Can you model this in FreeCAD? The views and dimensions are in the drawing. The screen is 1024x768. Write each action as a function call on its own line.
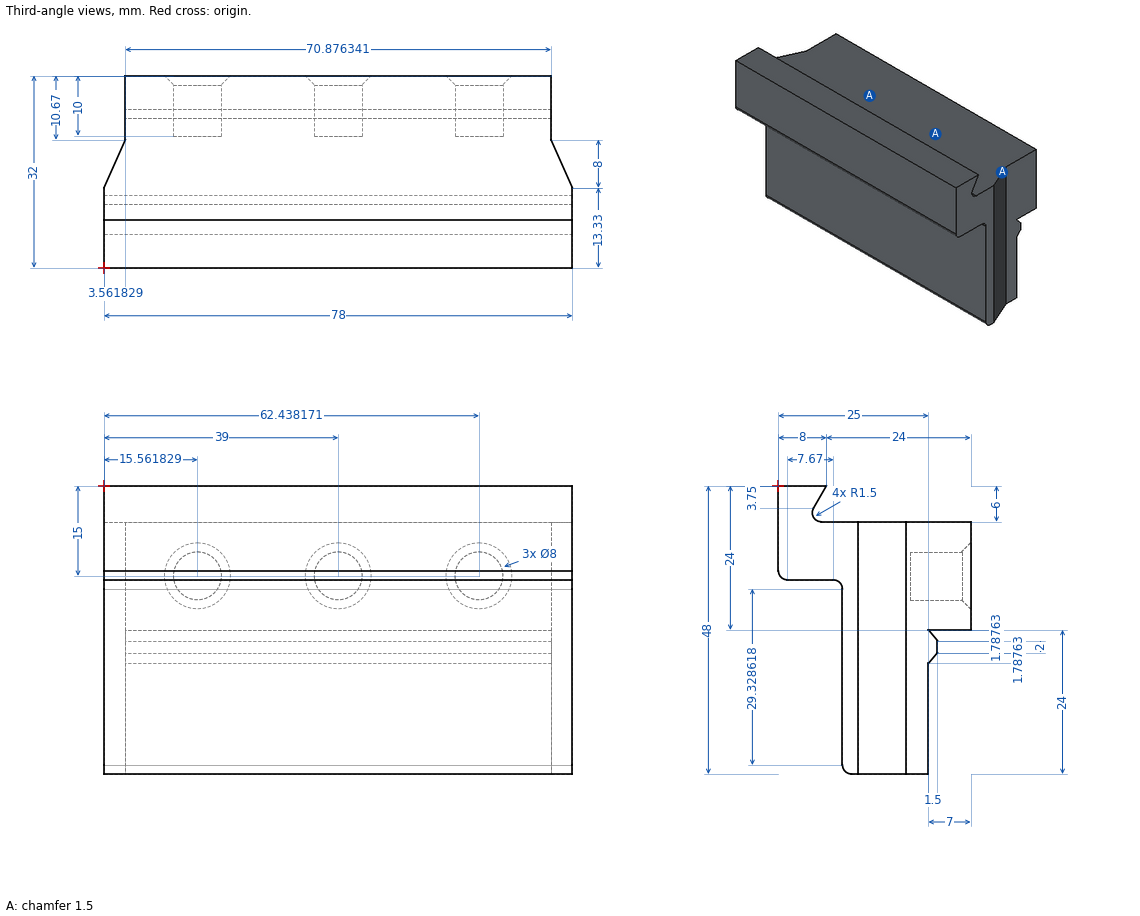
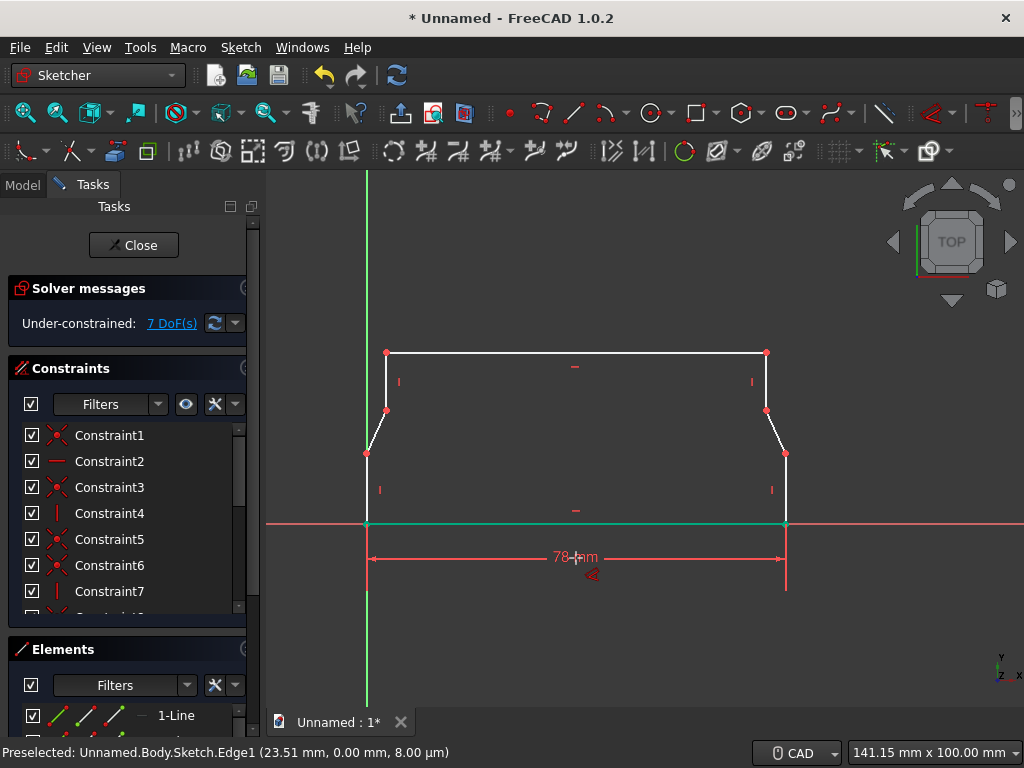
click(780, 441)
click(820, 433)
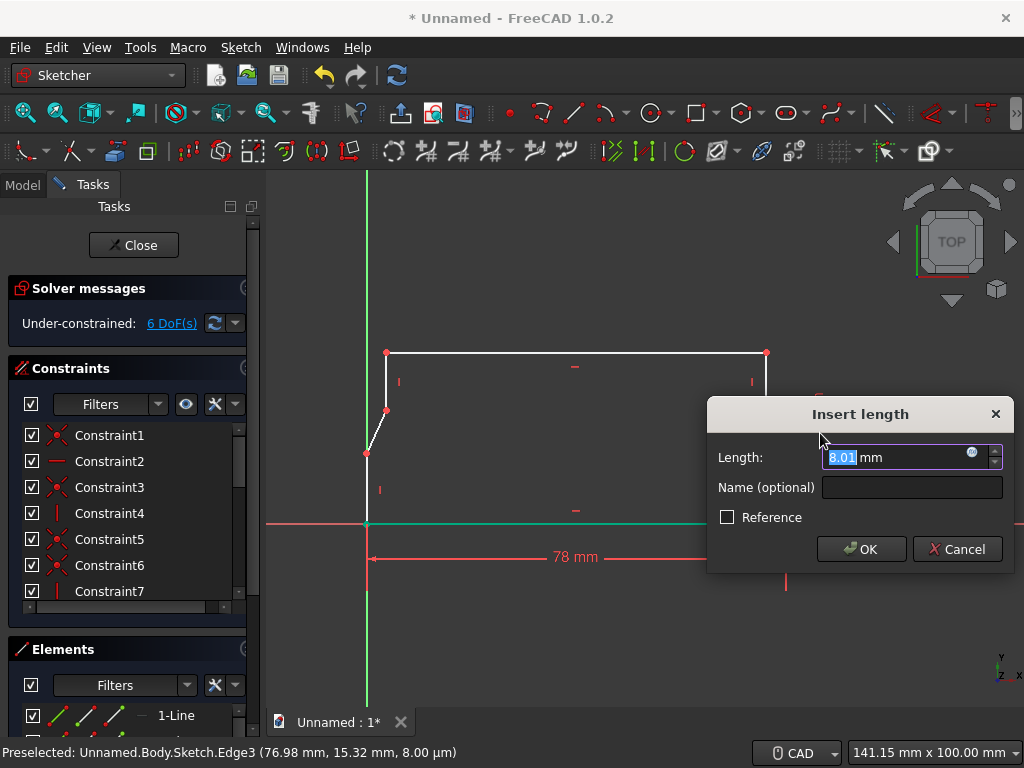
text(8)
key(Return)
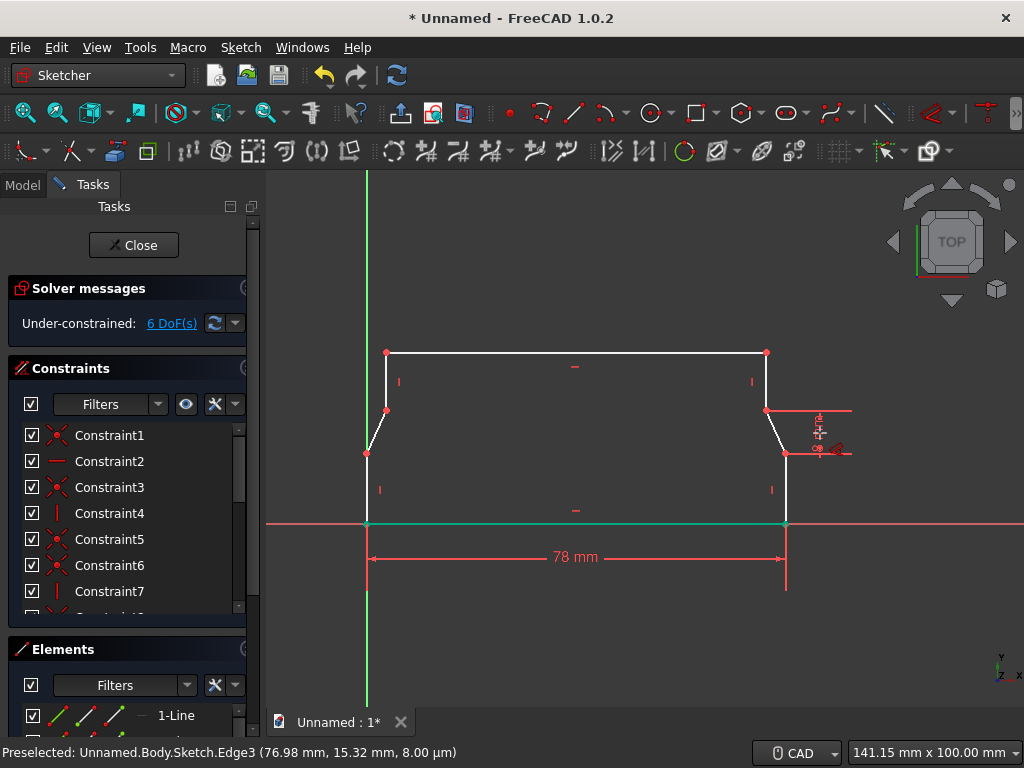
click(380, 424)
click(333, 433)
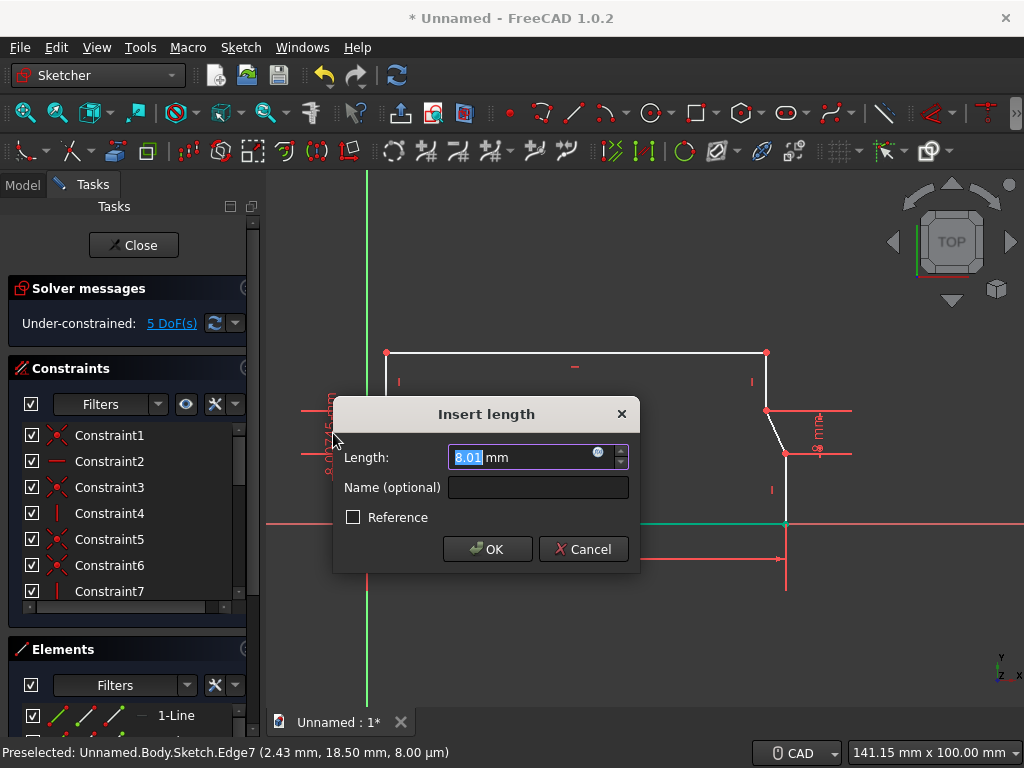
text(8)
key(Return)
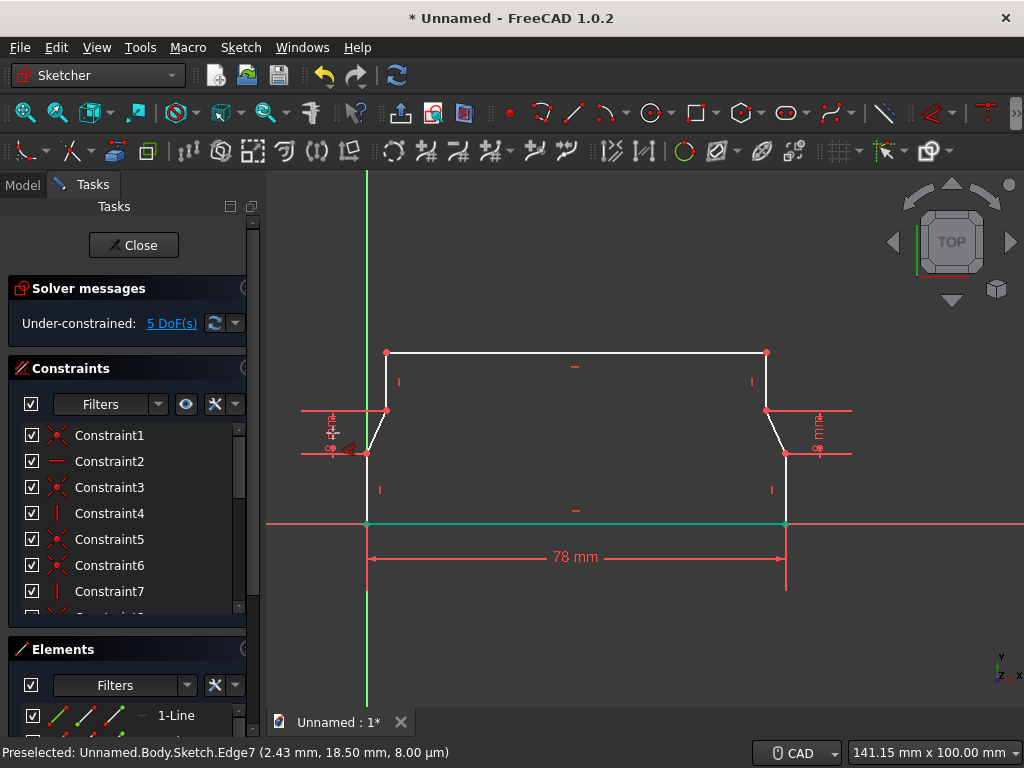
click(766, 353)
click(333, 399)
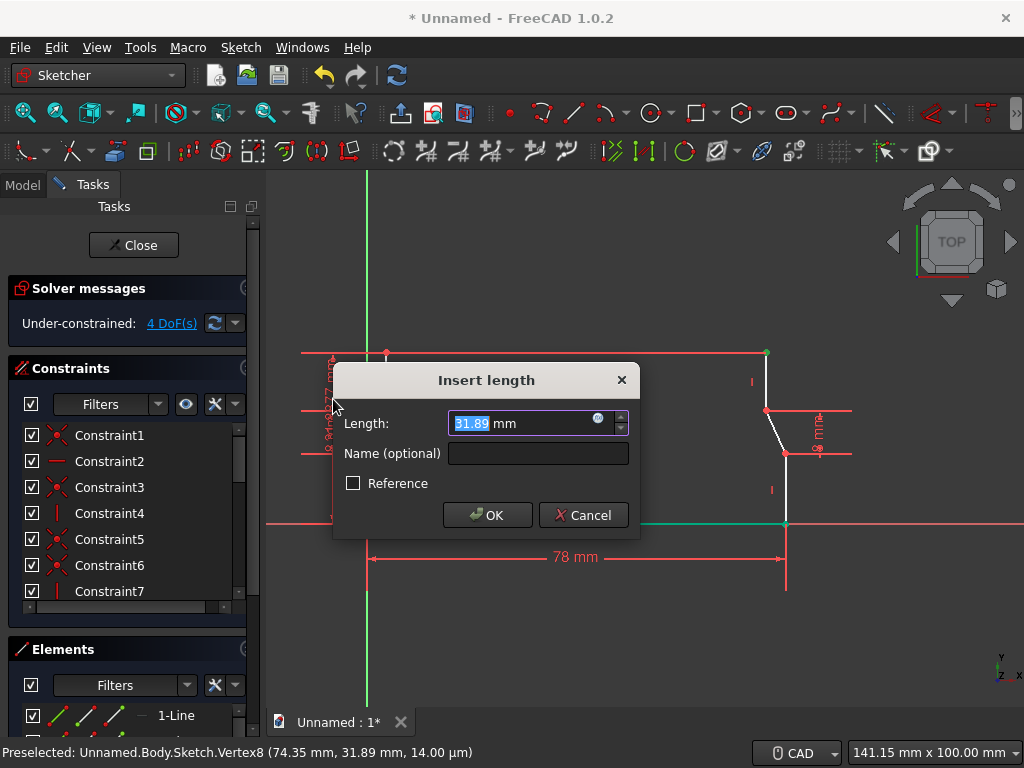
text(32)
key(Return)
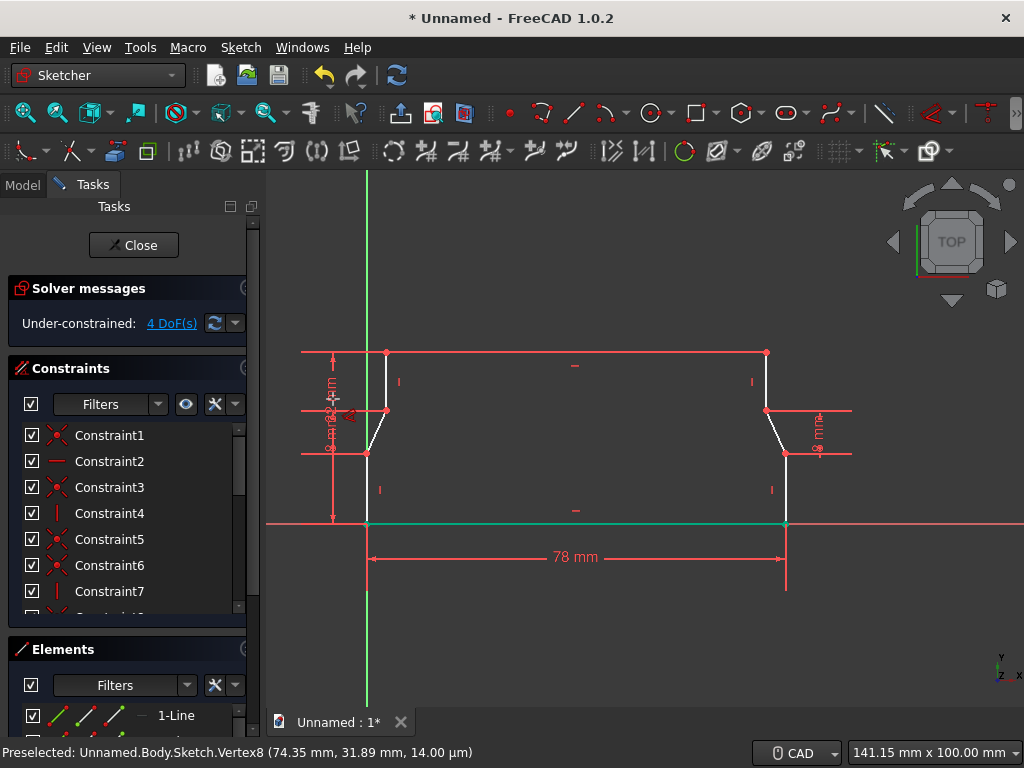
click(786, 503)
click(820, 489)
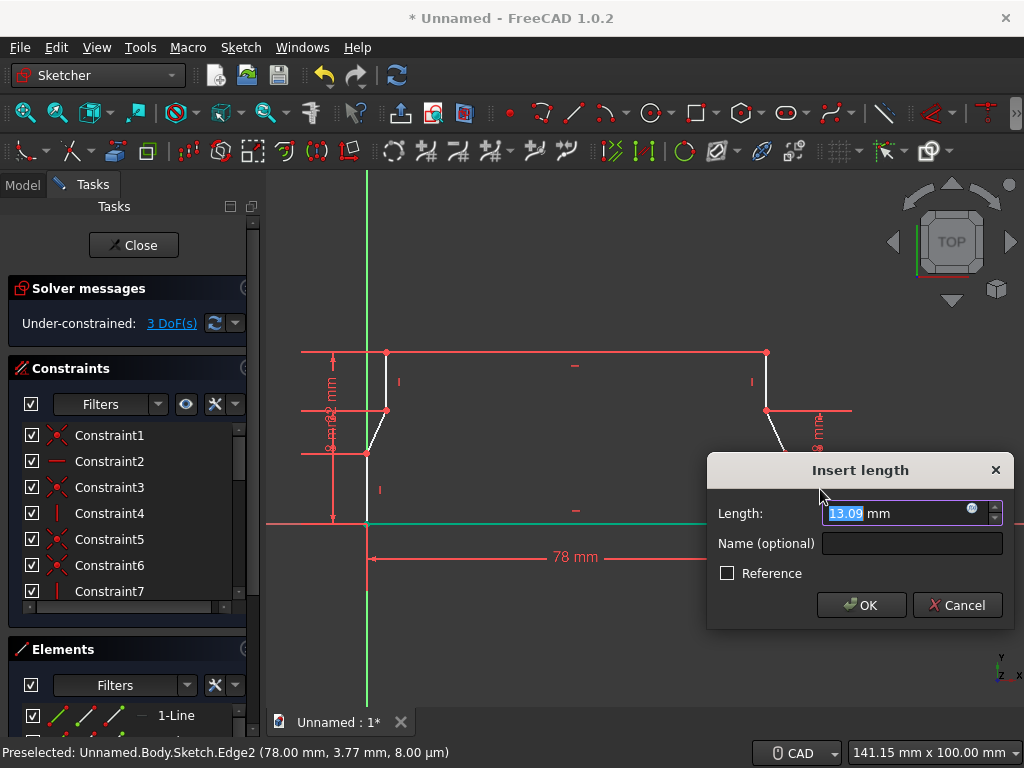
text(13.33)
key(Return)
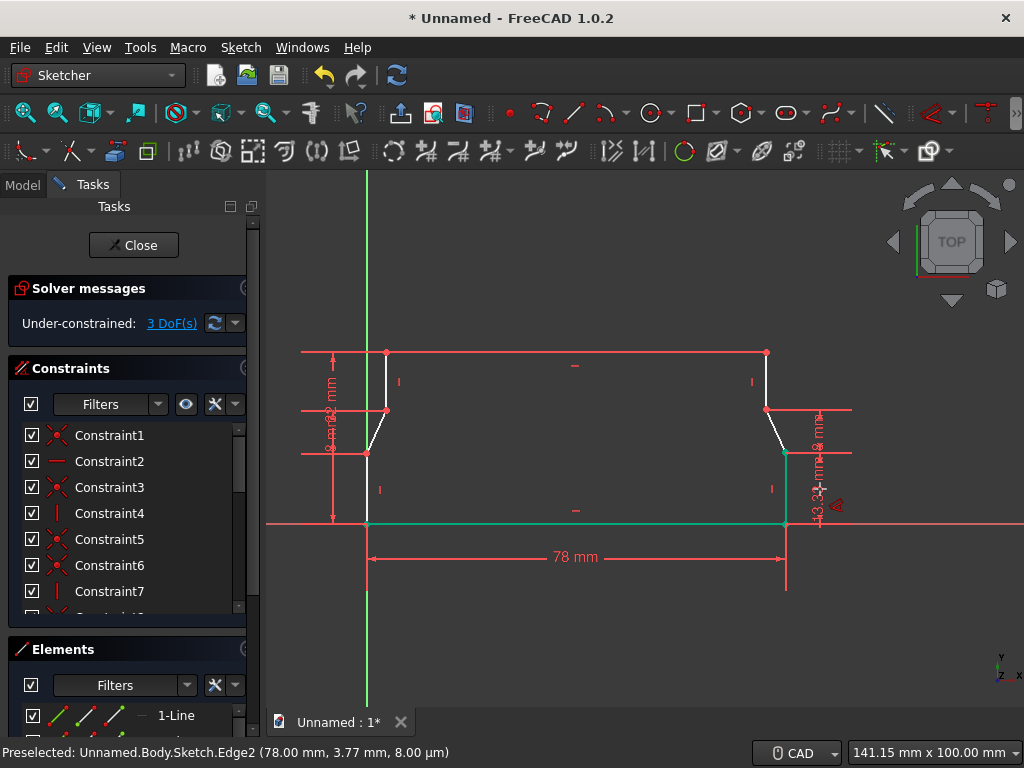
click(386, 370)
click(352, 368)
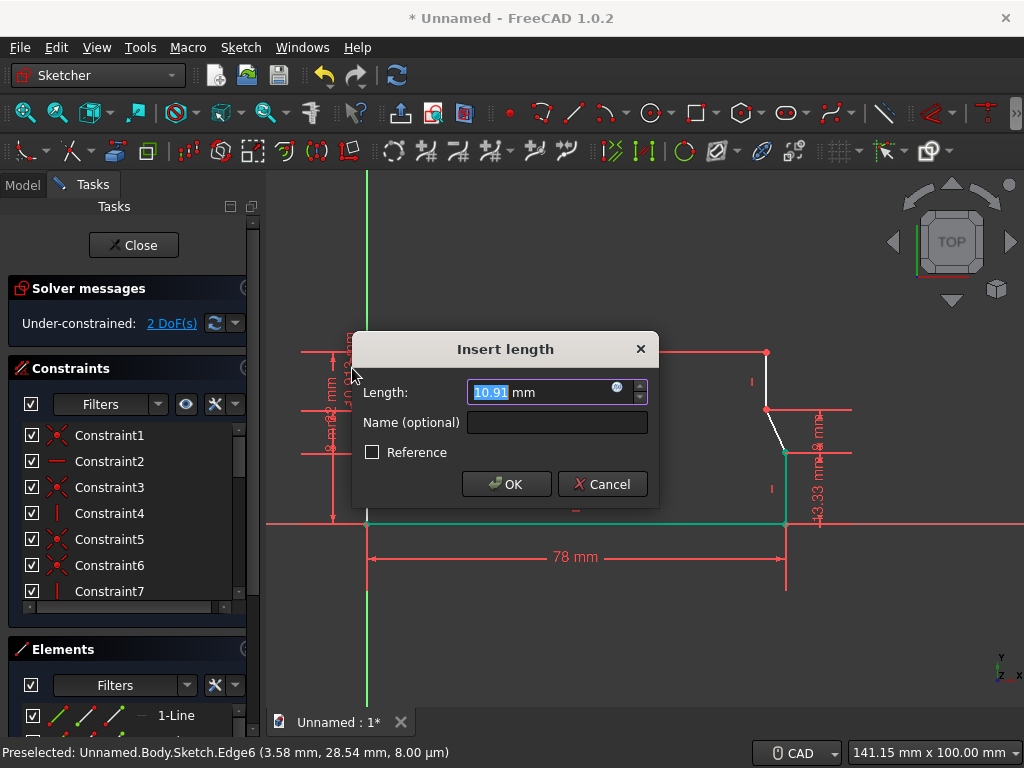
text(10.67)
key(Return)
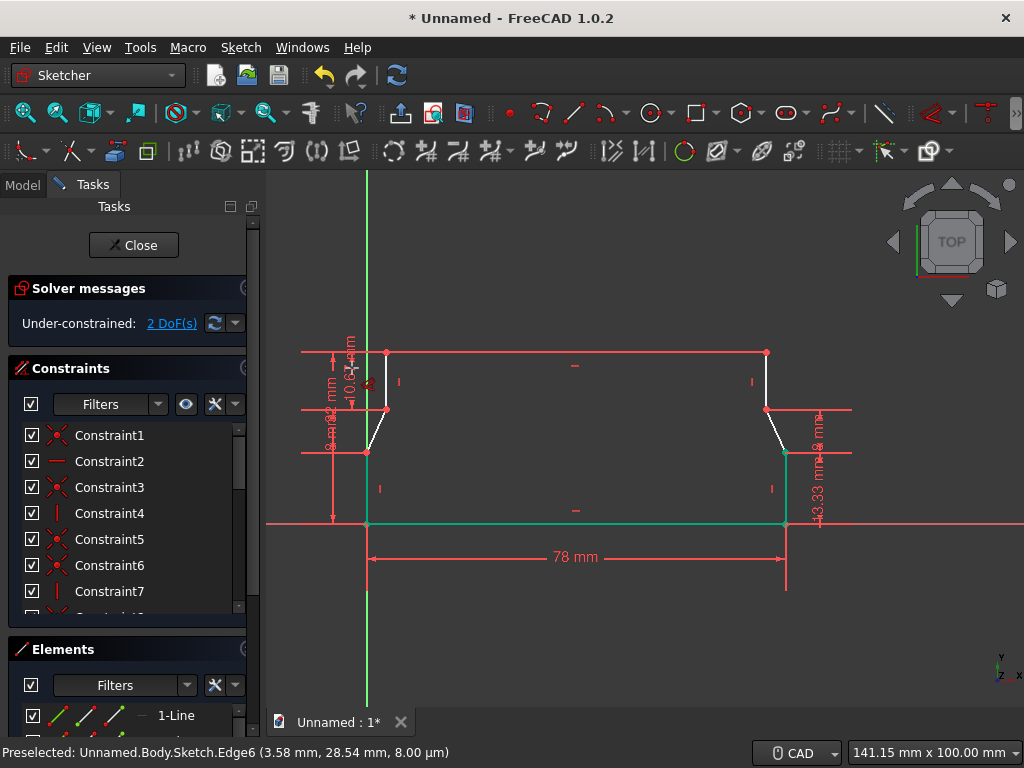
click(652, 352)
click(576, 318)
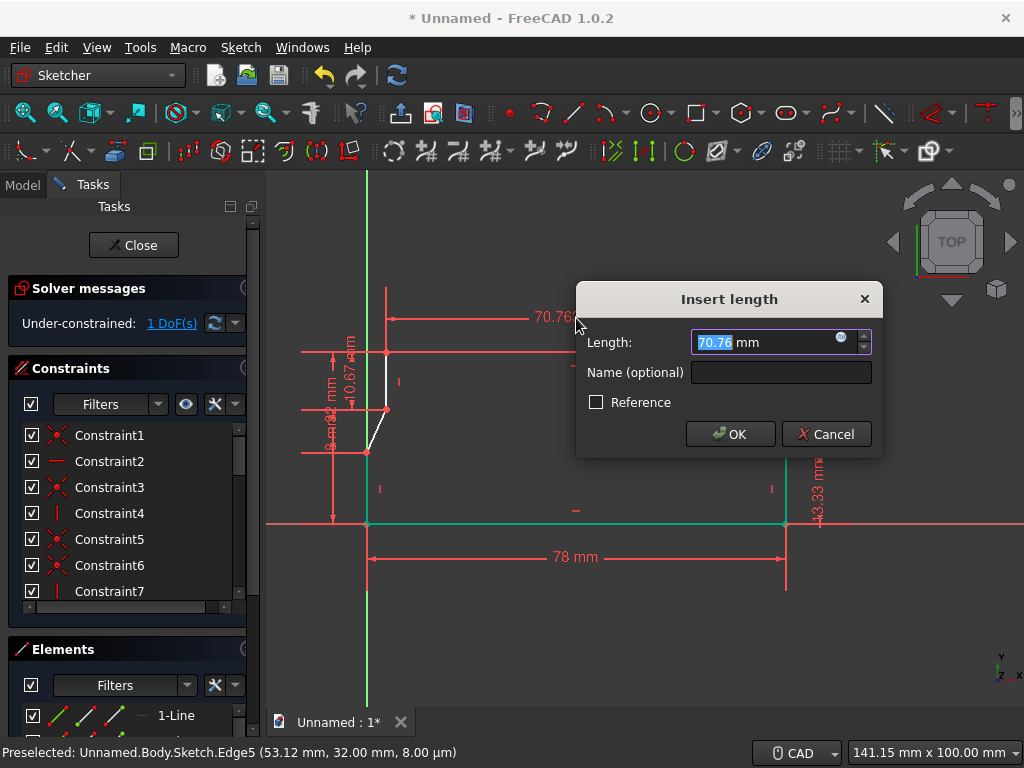
text(70.876341)
key(Return)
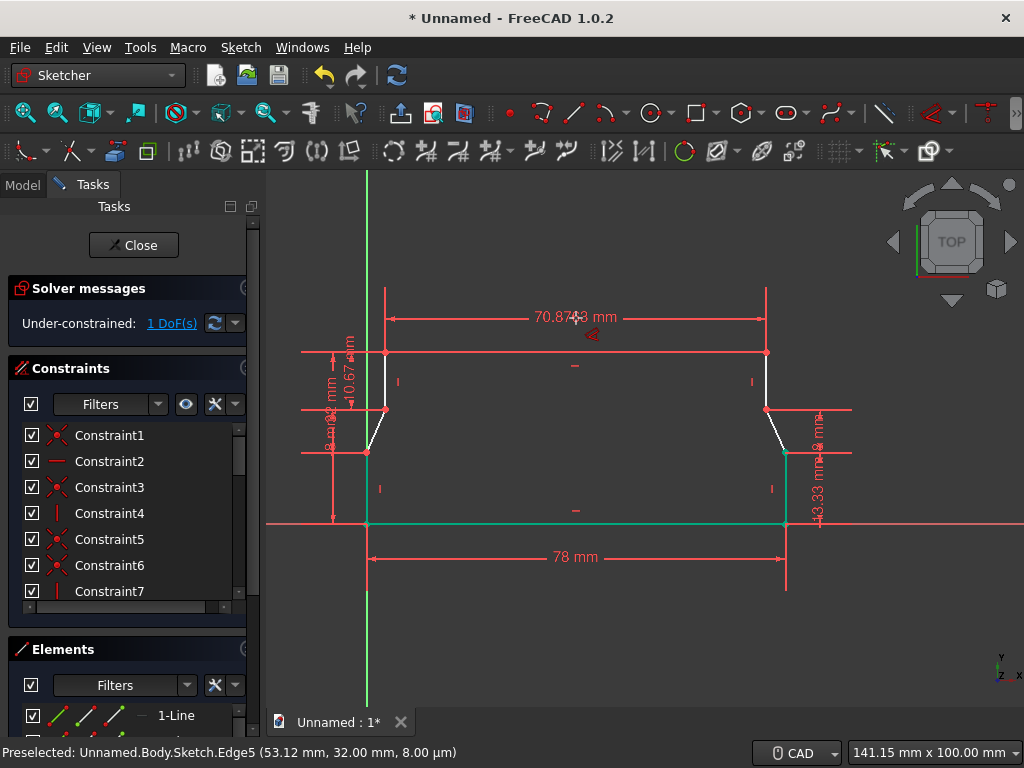
scroll(385, 352, up, 4)